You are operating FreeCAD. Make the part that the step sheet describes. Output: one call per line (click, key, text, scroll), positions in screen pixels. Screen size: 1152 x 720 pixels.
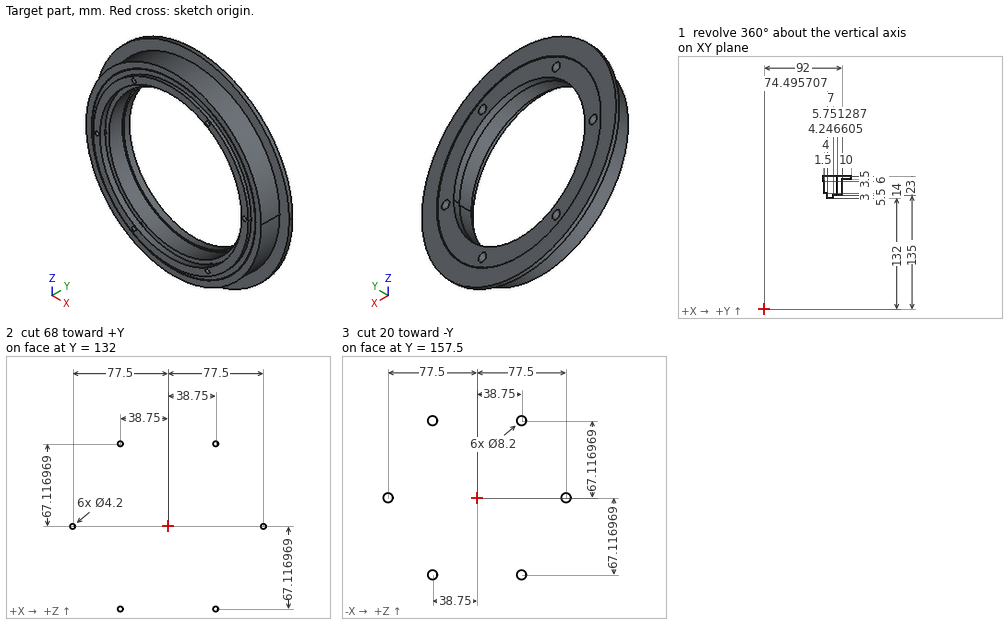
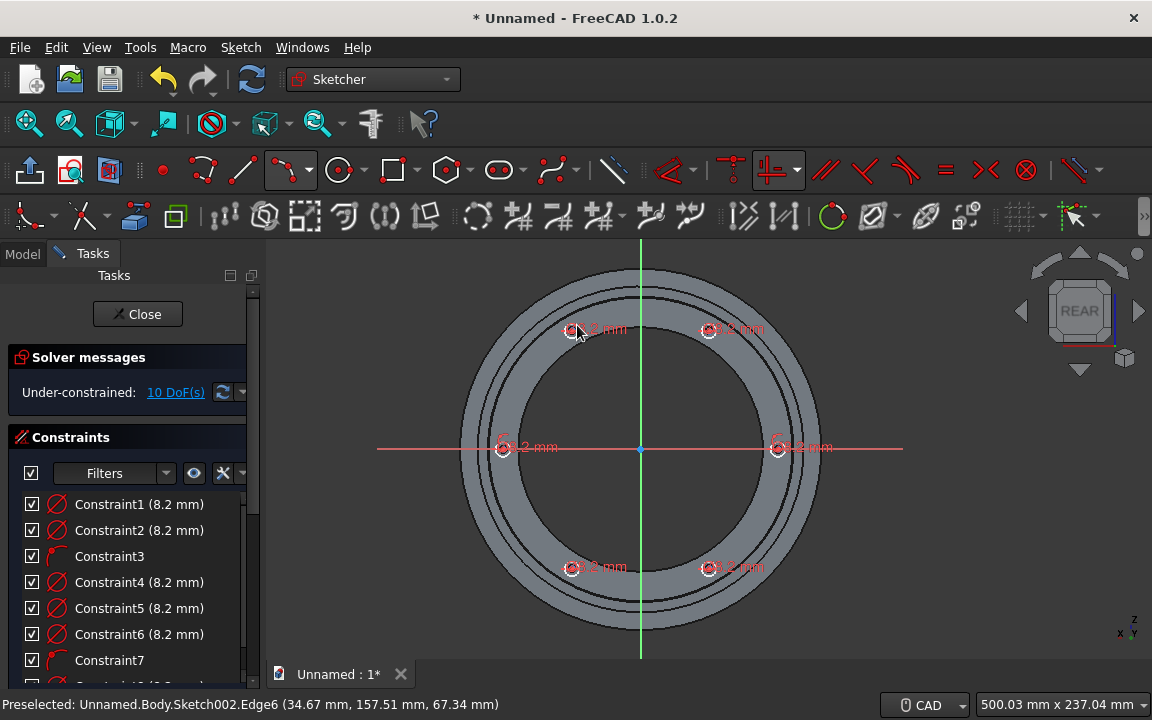
click(709, 331)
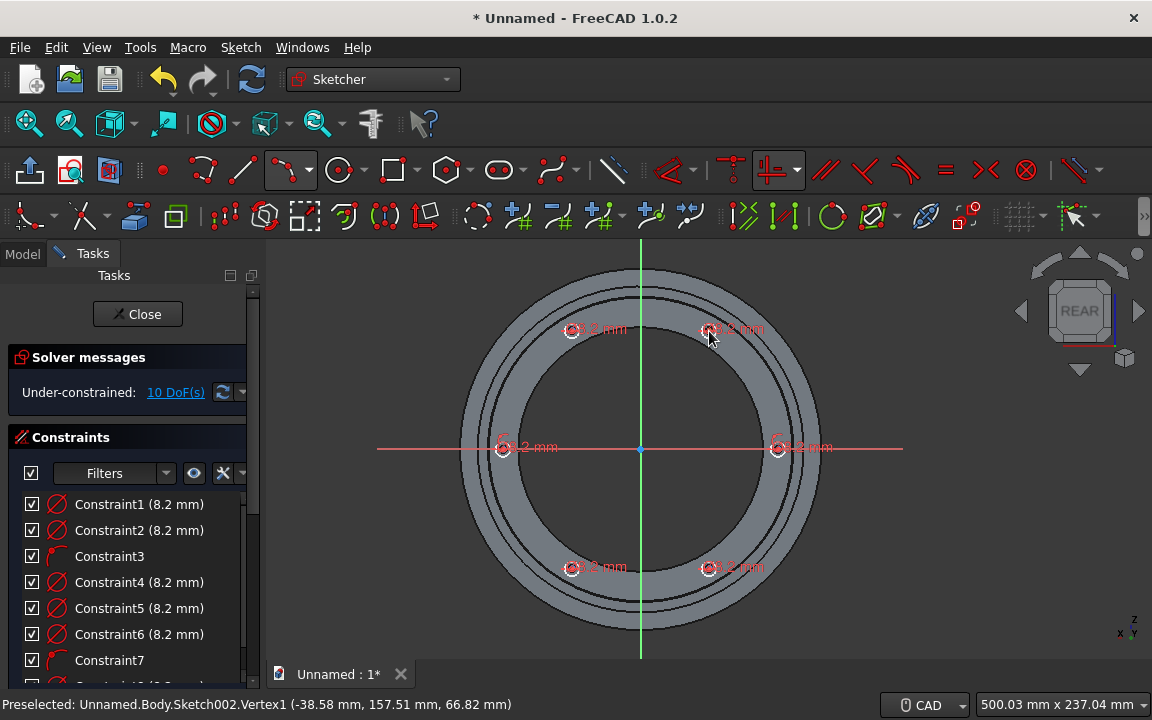
click(709, 569)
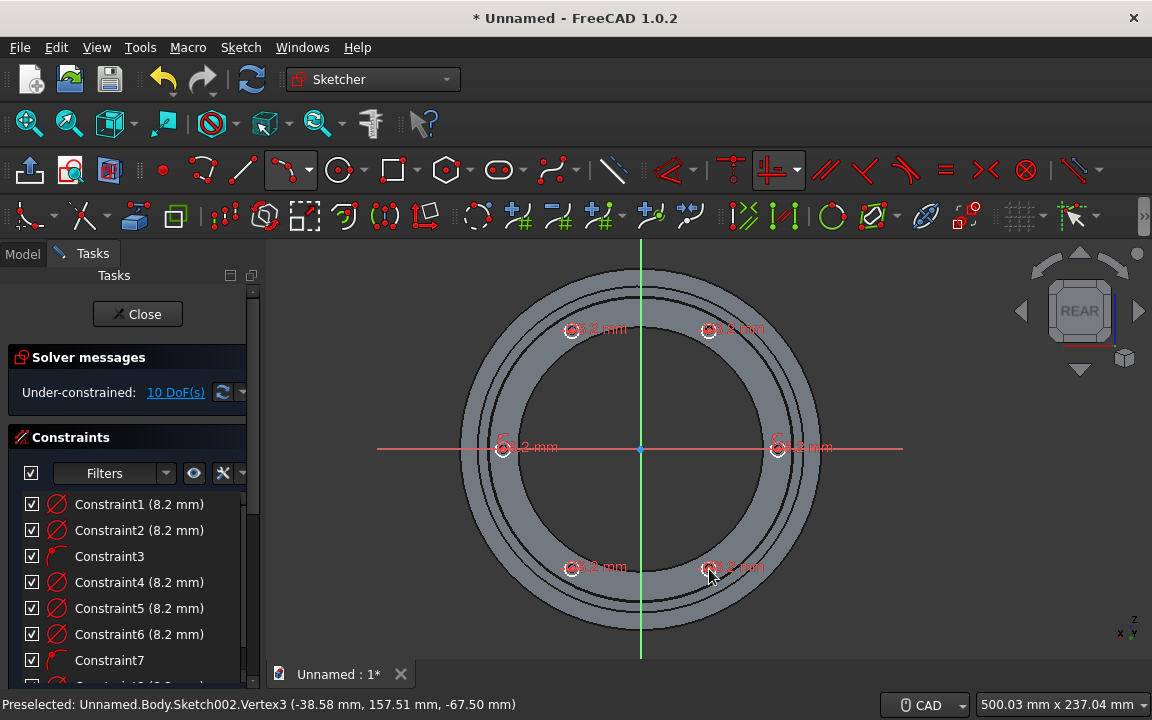
click(800, 170)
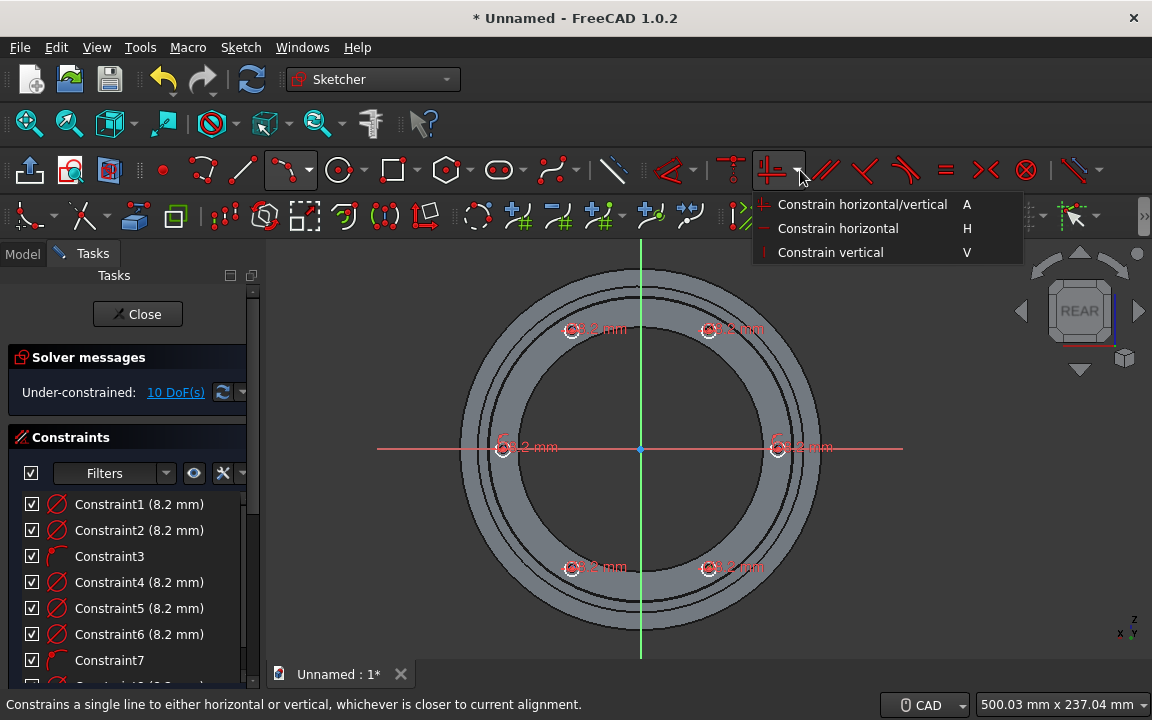
click(888, 252)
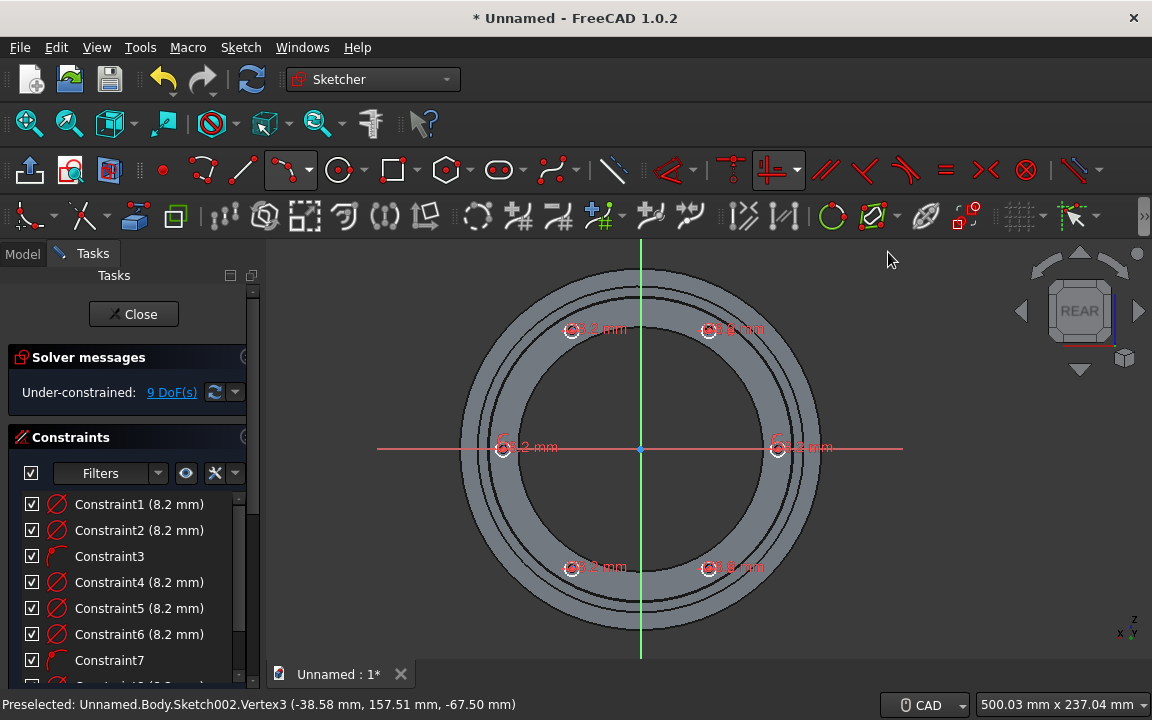
click(709, 569)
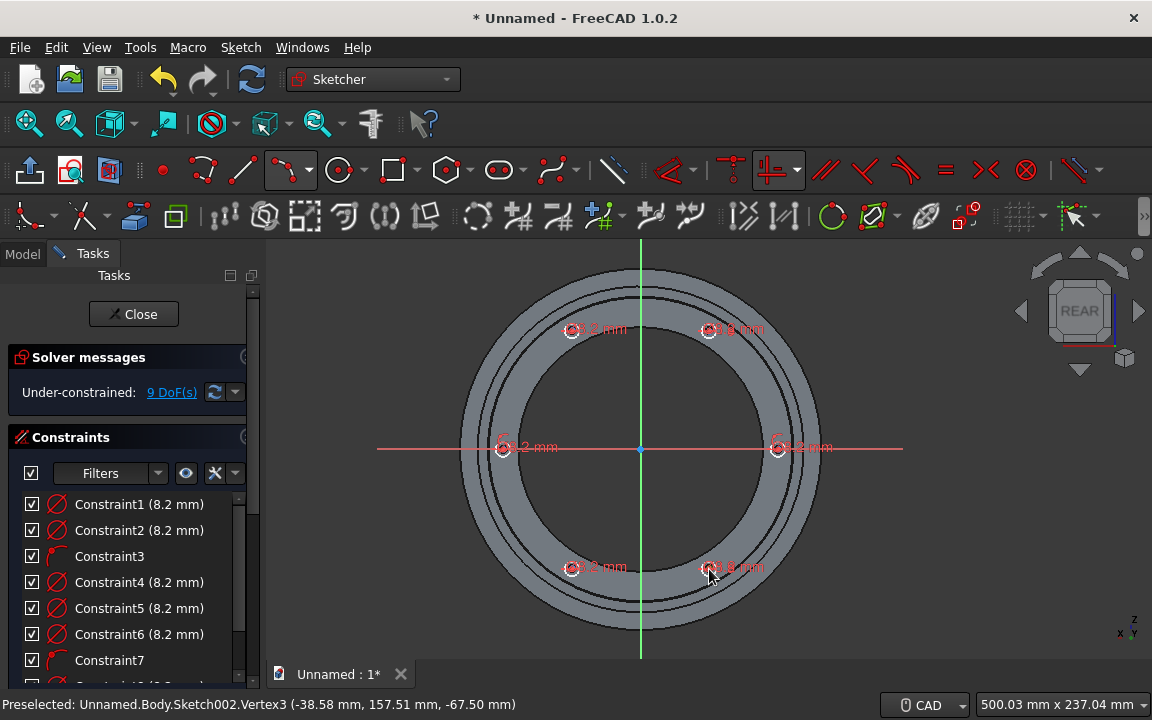
click(572, 569)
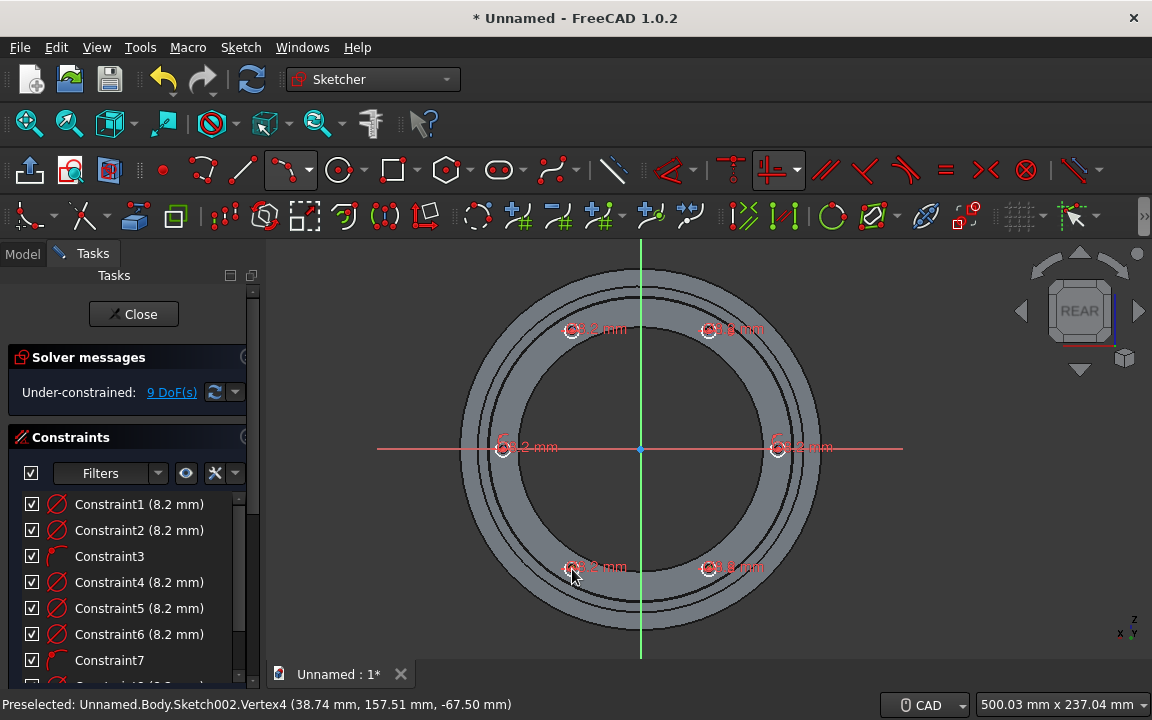
click(800, 170)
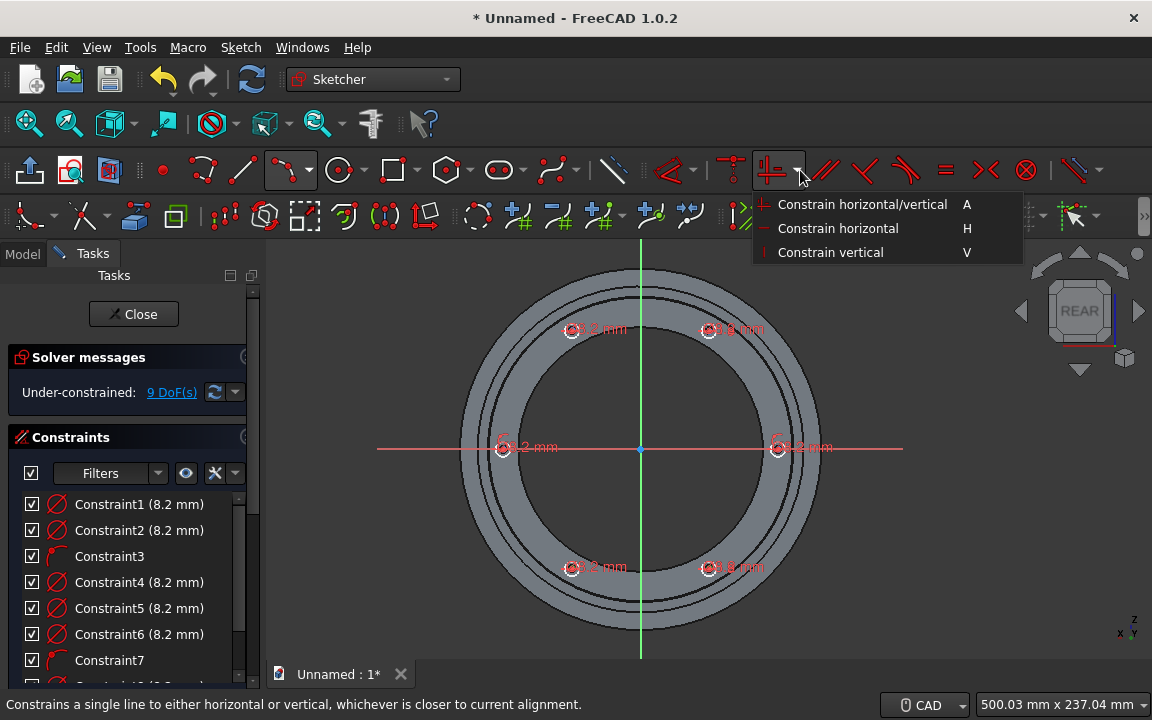
click(888, 228)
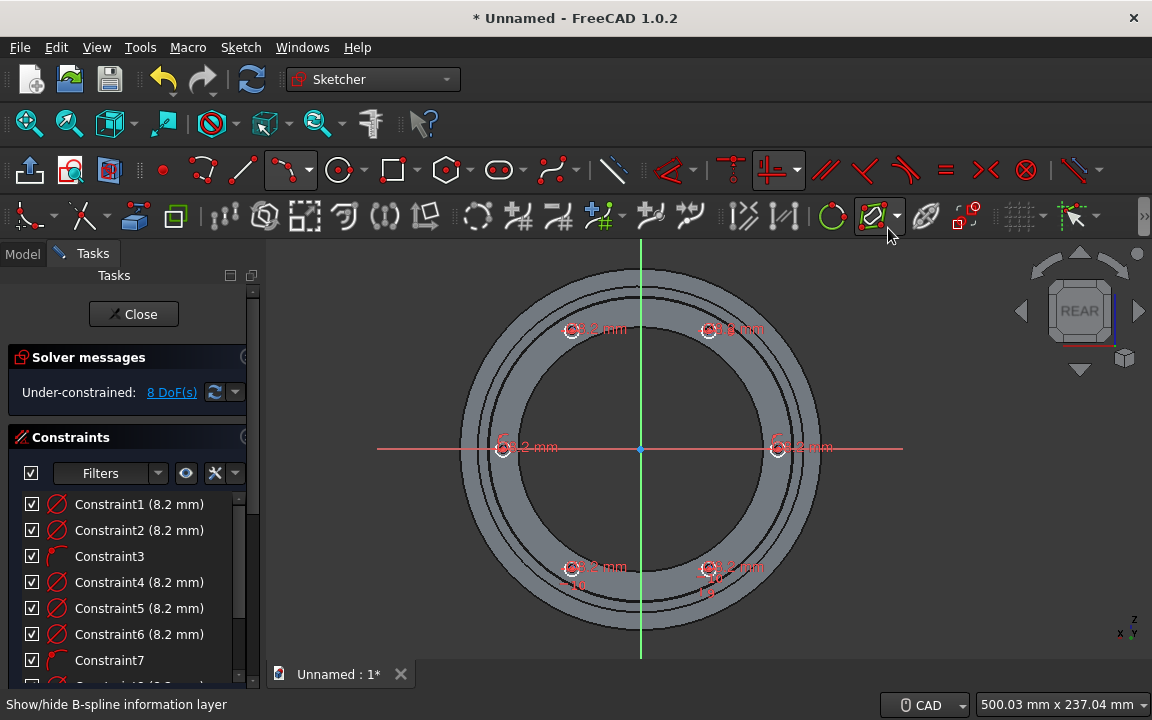
click(572, 569)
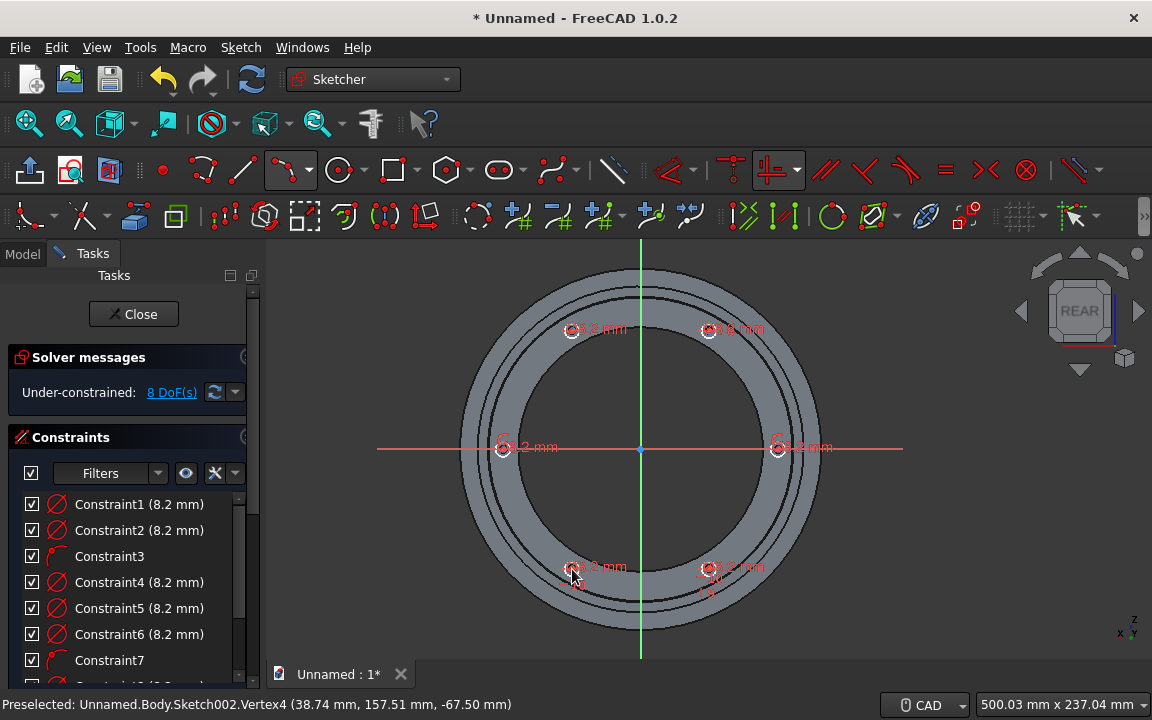
click(572, 331)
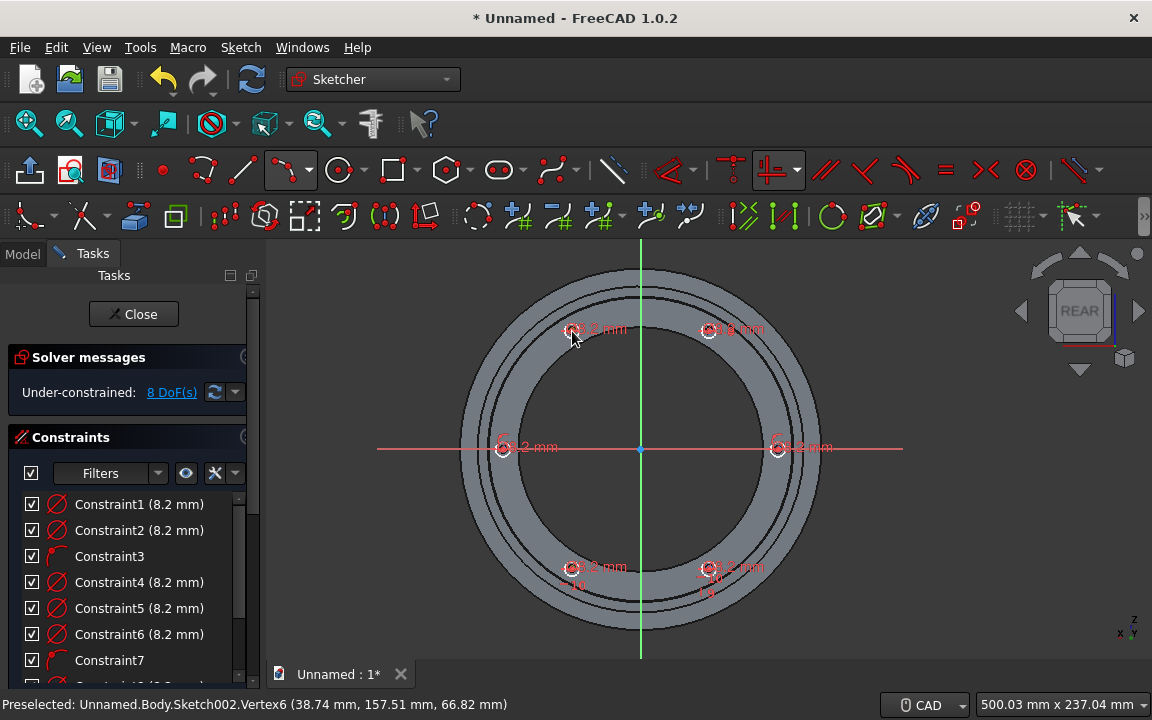
key(v)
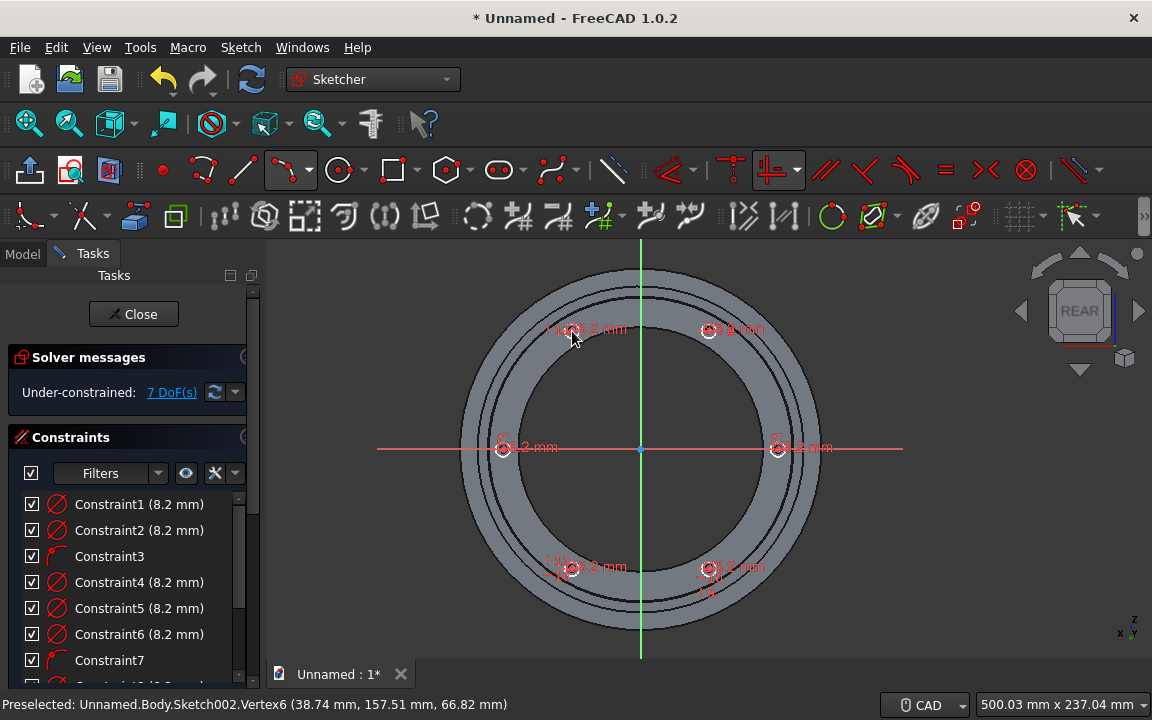
click(709, 331)